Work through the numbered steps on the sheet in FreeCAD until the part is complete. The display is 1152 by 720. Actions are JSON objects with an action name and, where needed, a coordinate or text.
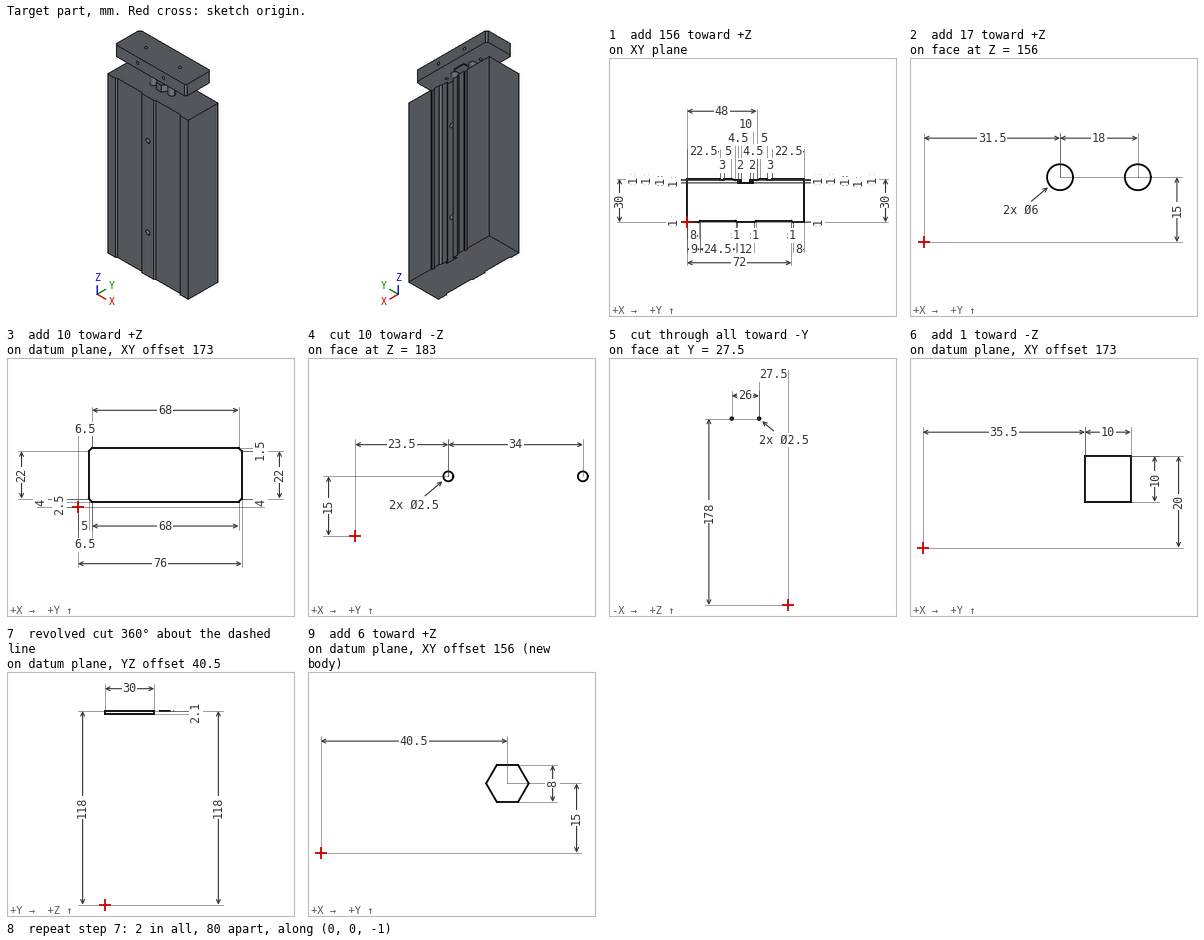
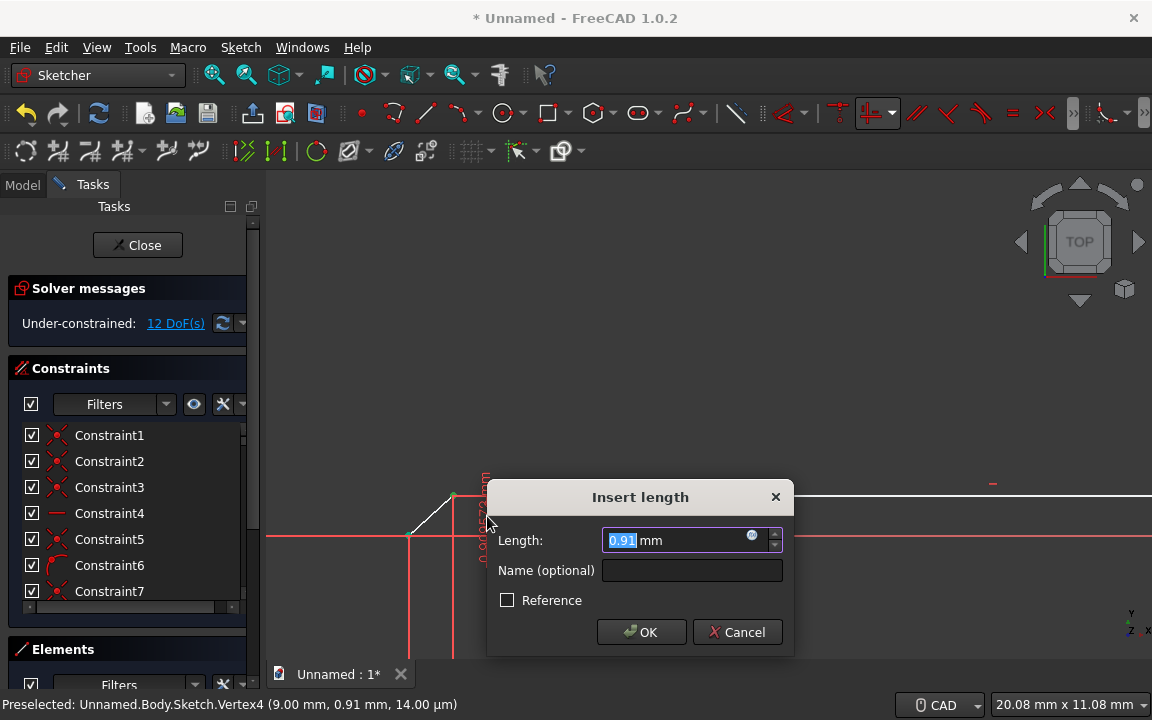
{"action": "type", "text": "1"}
{"action": "key", "text": "Return"}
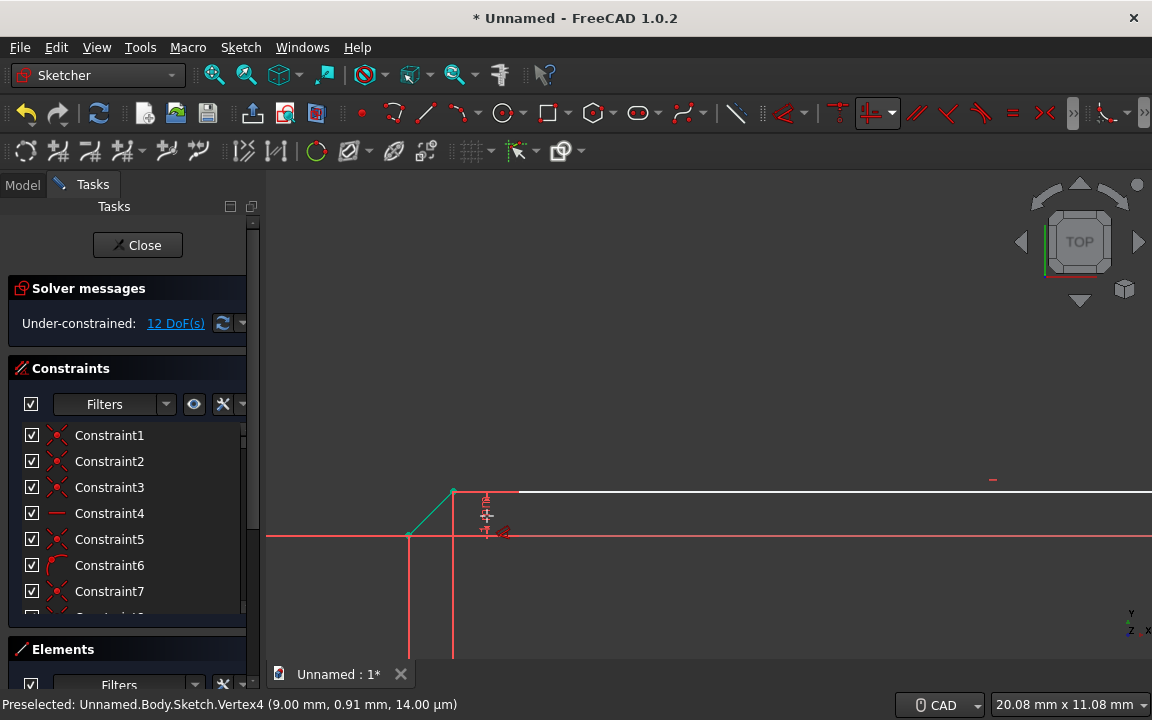
{"action": "scroll", "coordinate": [452, 499], "scroll_direction": "down", "scroll_amount": 10}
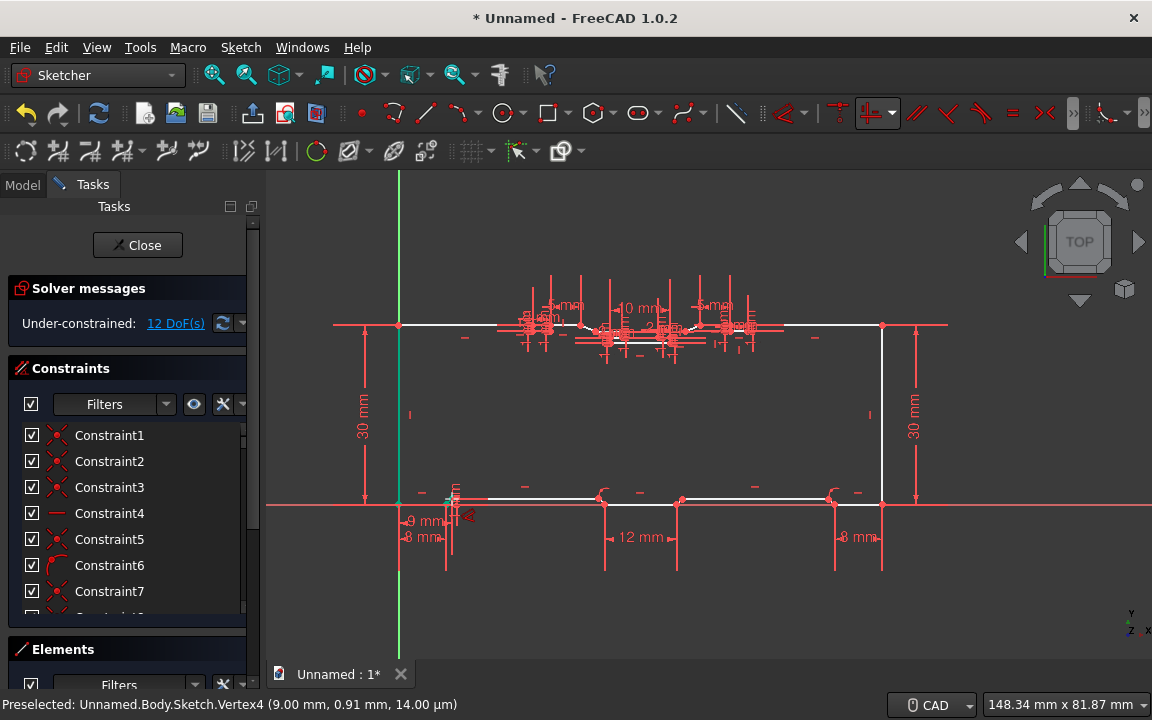
{"action": "scroll", "coordinate": [682, 499], "scroll_direction": "up", "scroll_amount": 10}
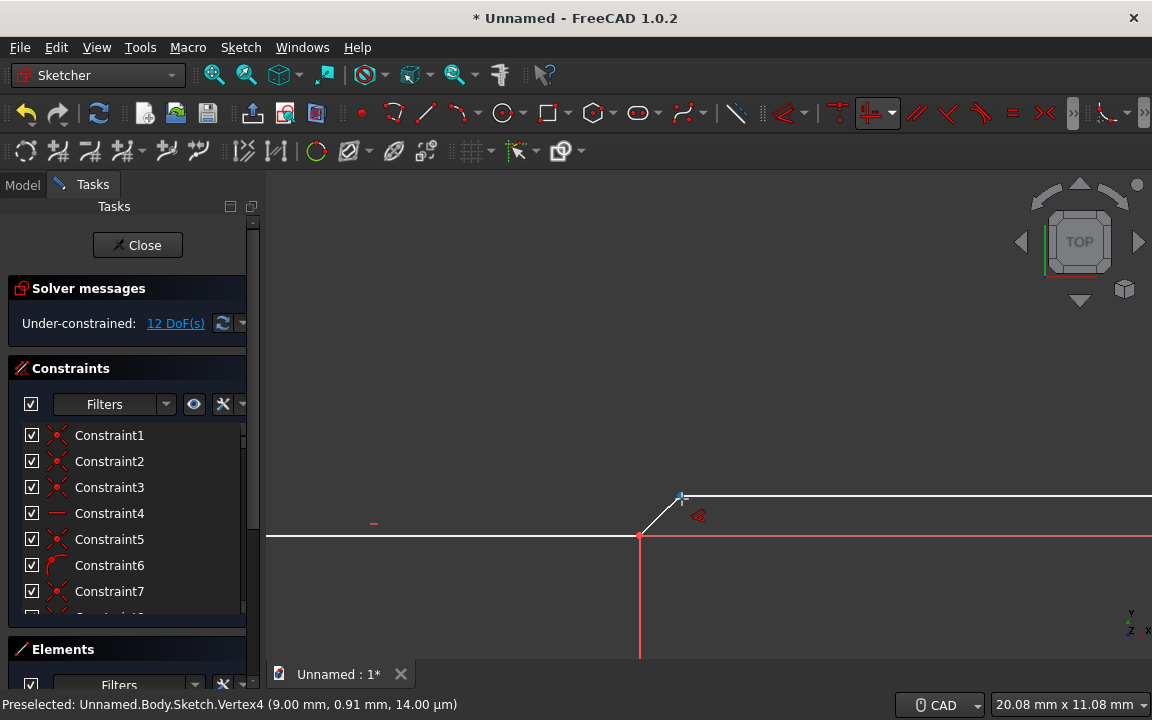
{"action": "left_click", "coordinate": [681, 496]}
{"action": "left_click", "coordinate": [715, 516]}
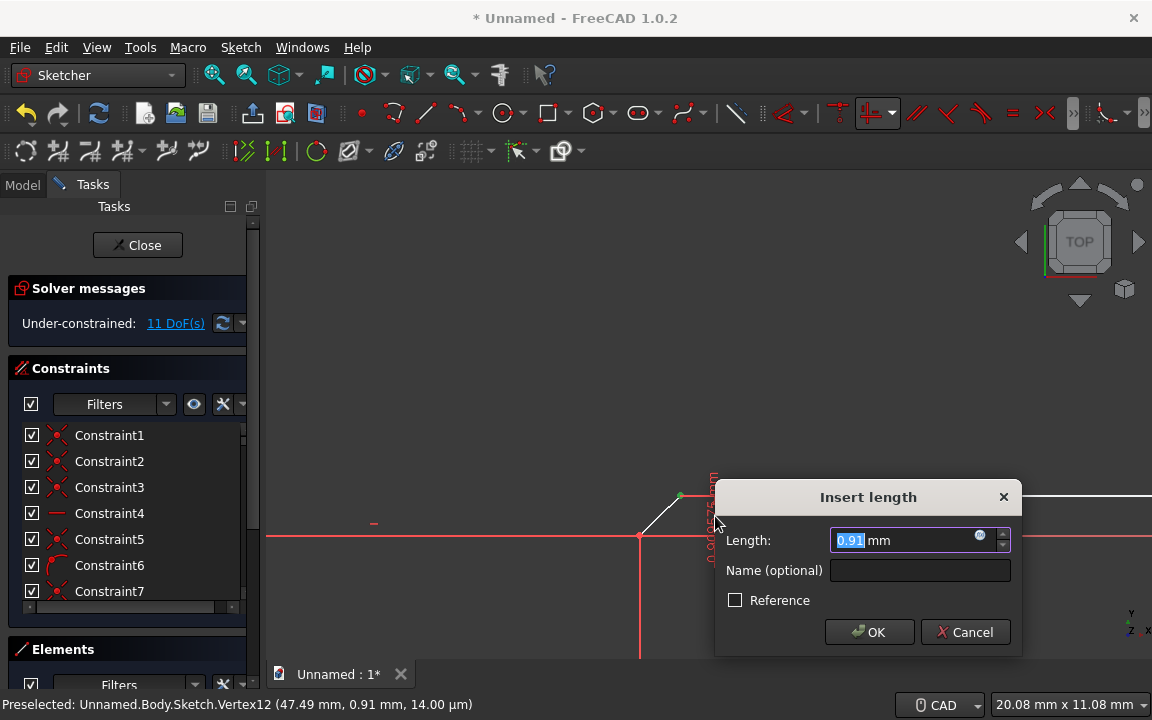
{"action": "type", "text": "1"}
{"action": "key", "text": "Return"}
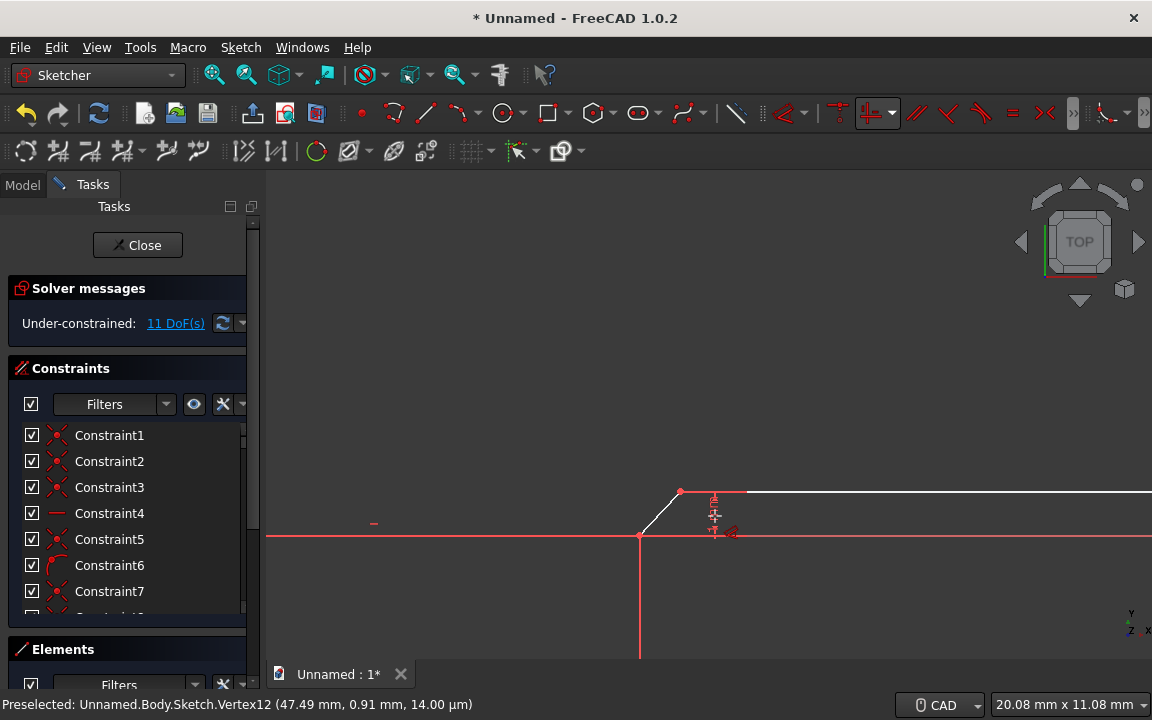
{"action": "scroll", "coordinate": [683, 499], "scroll_direction": "down", "scroll_amount": 10}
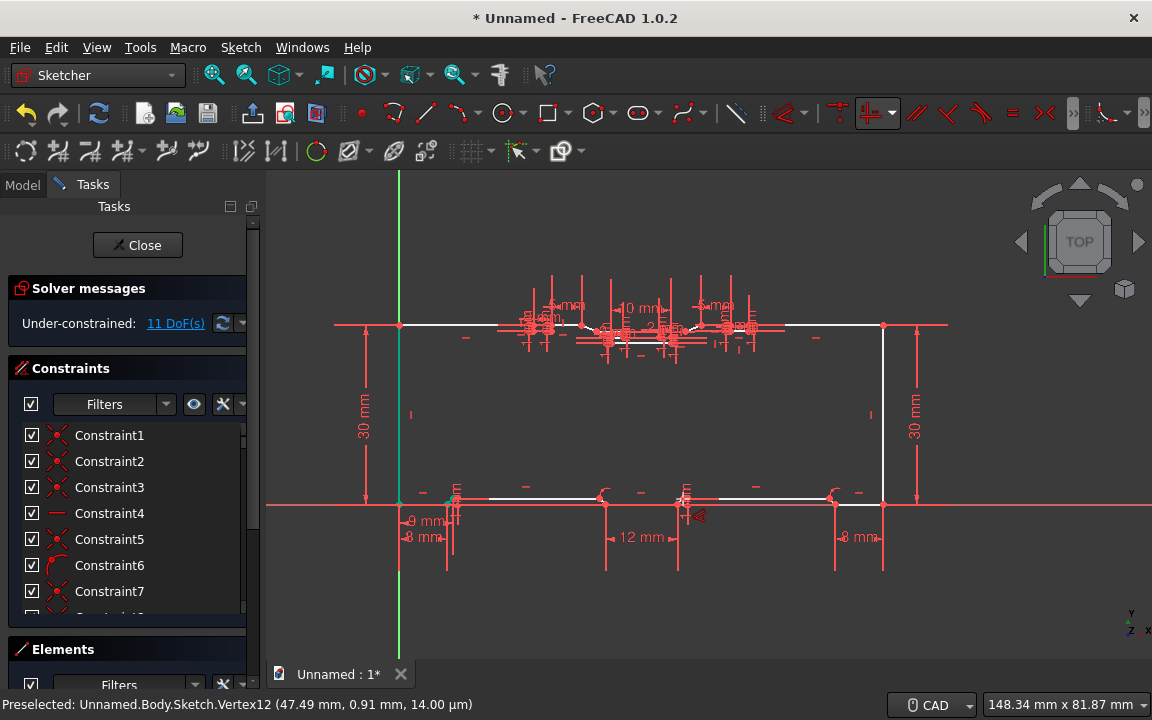
{"action": "scroll", "coordinate": [601, 500], "scroll_direction": "up", "scroll_amount": 10}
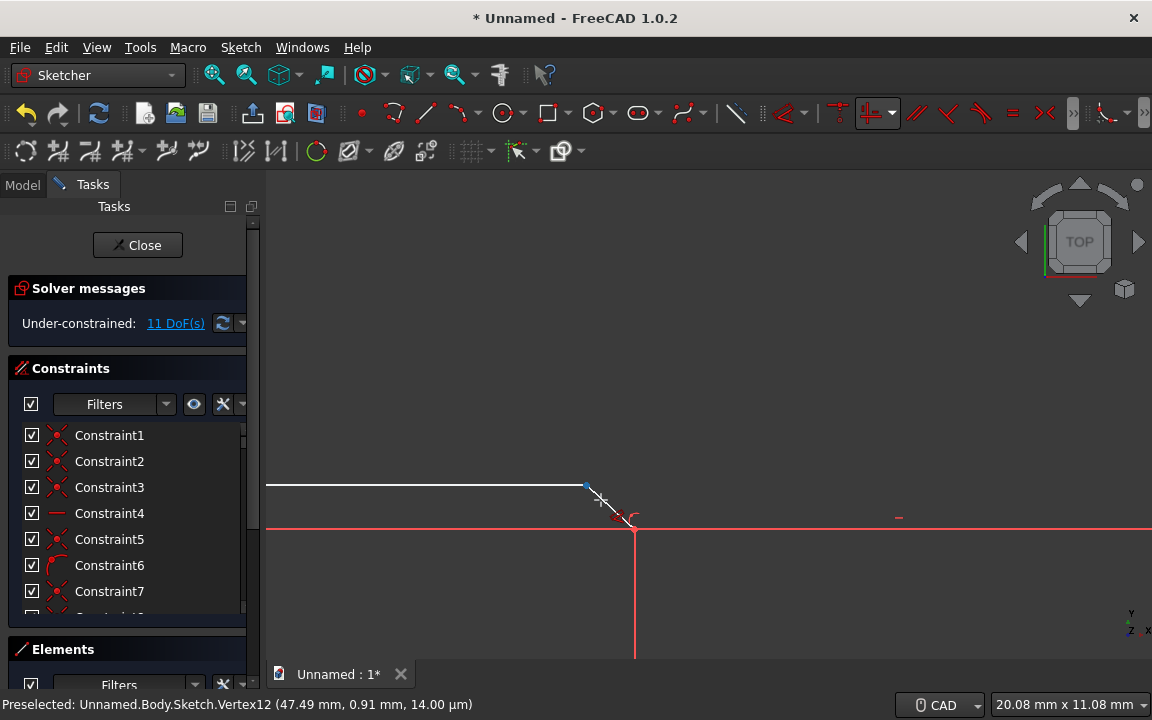
{"action": "left_click", "coordinate": [601, 498]}
{"action": "left_click", "coordinate": [611, 563]}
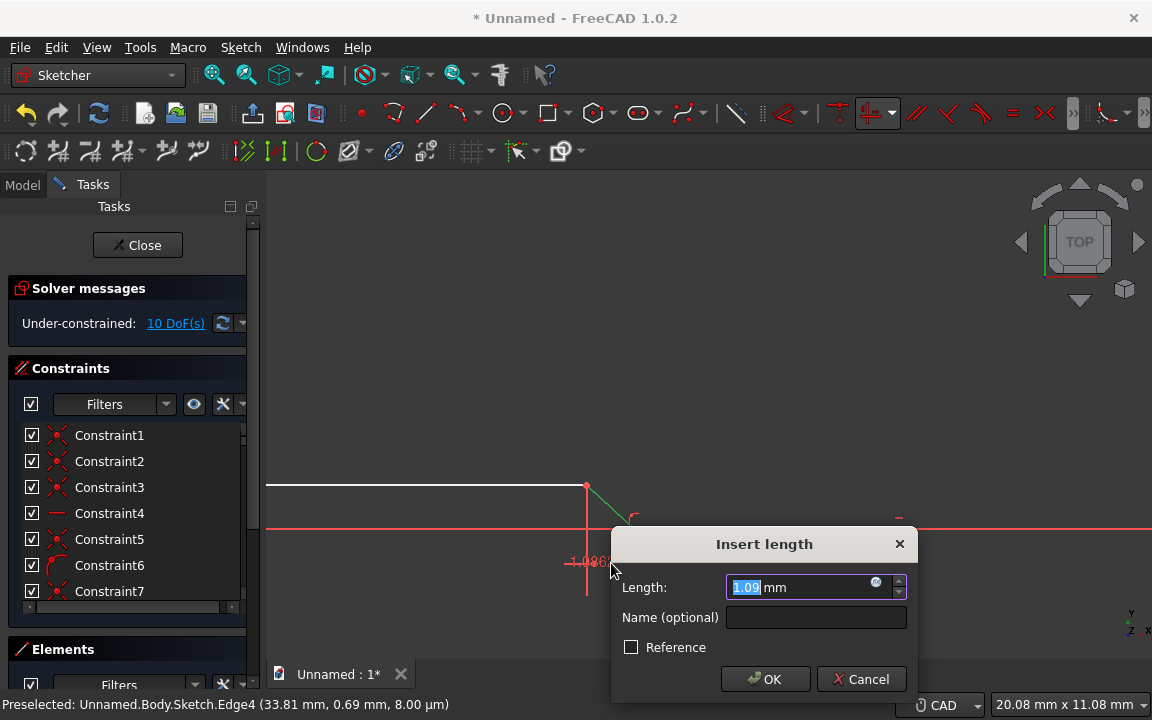
{"action": "type", "text": "1"}
{"action": "key", "text": "Return"}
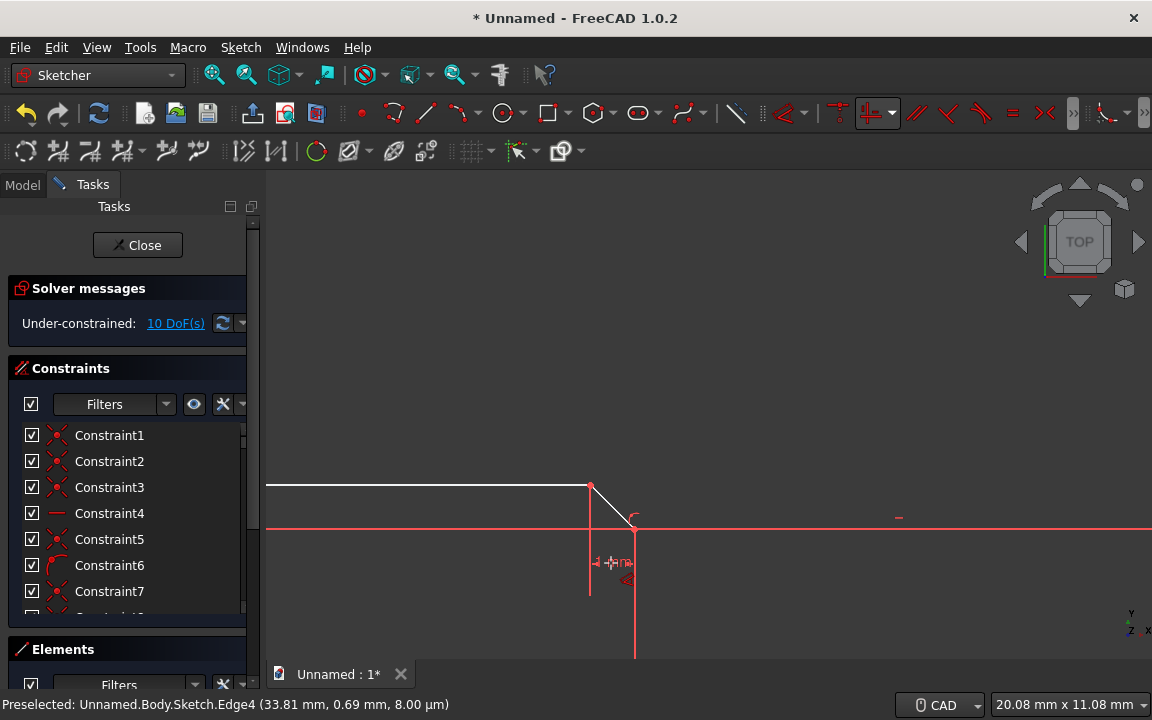
{"action": "scroll", "coordinate": [600, 500], "scroll_direction": "down", "scroll_amount": 10}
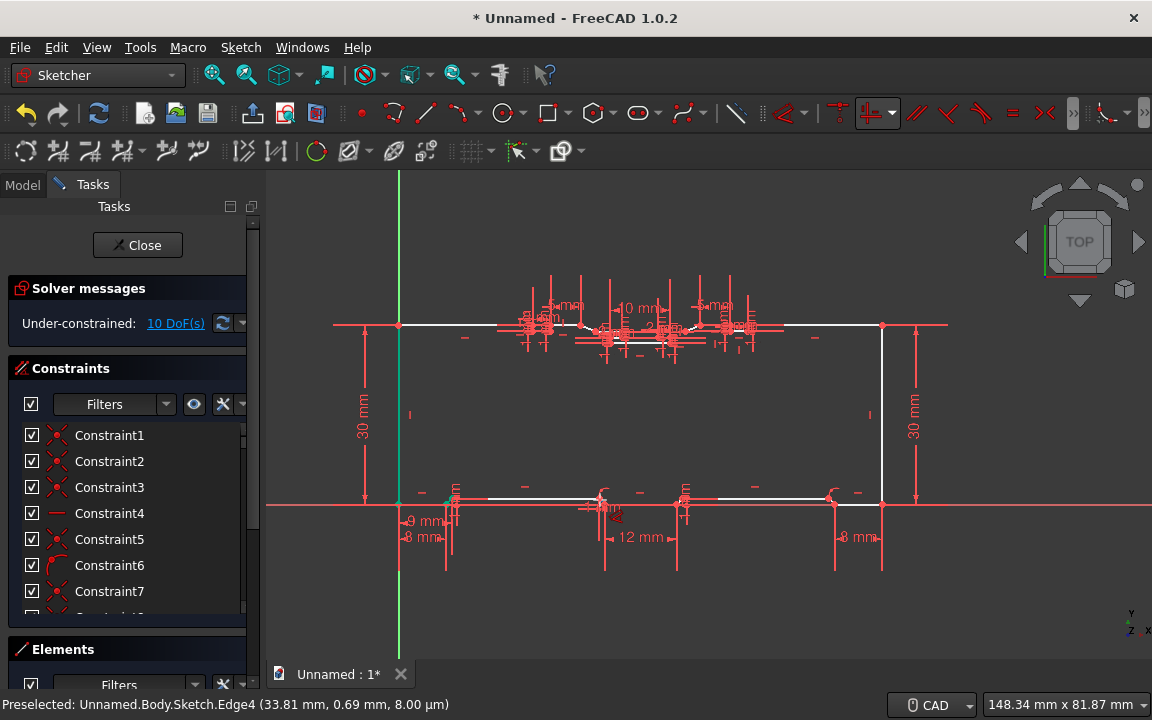
{"action": "scroll", "coordinate": [678, 503], "scroll_direction": "up", "scroll_amount": 11}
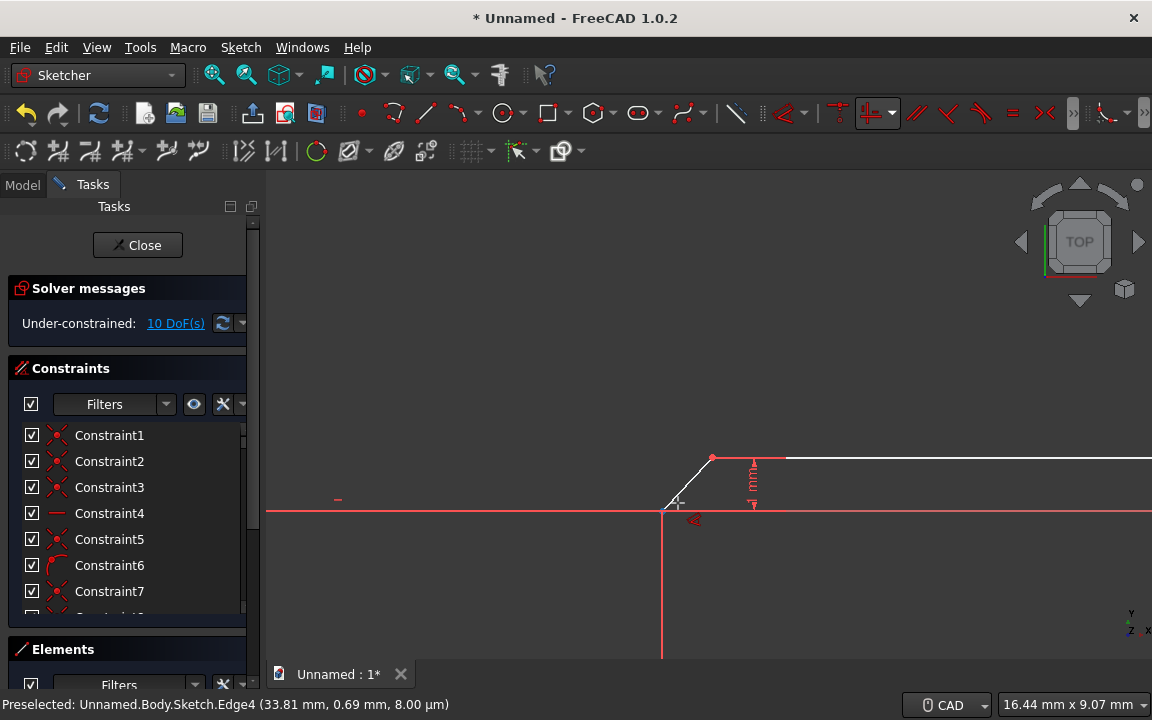
{"action": "left_click", "coordinate": [677, 495]}
{"action": "left_click", "coordinate": [687, 545]}